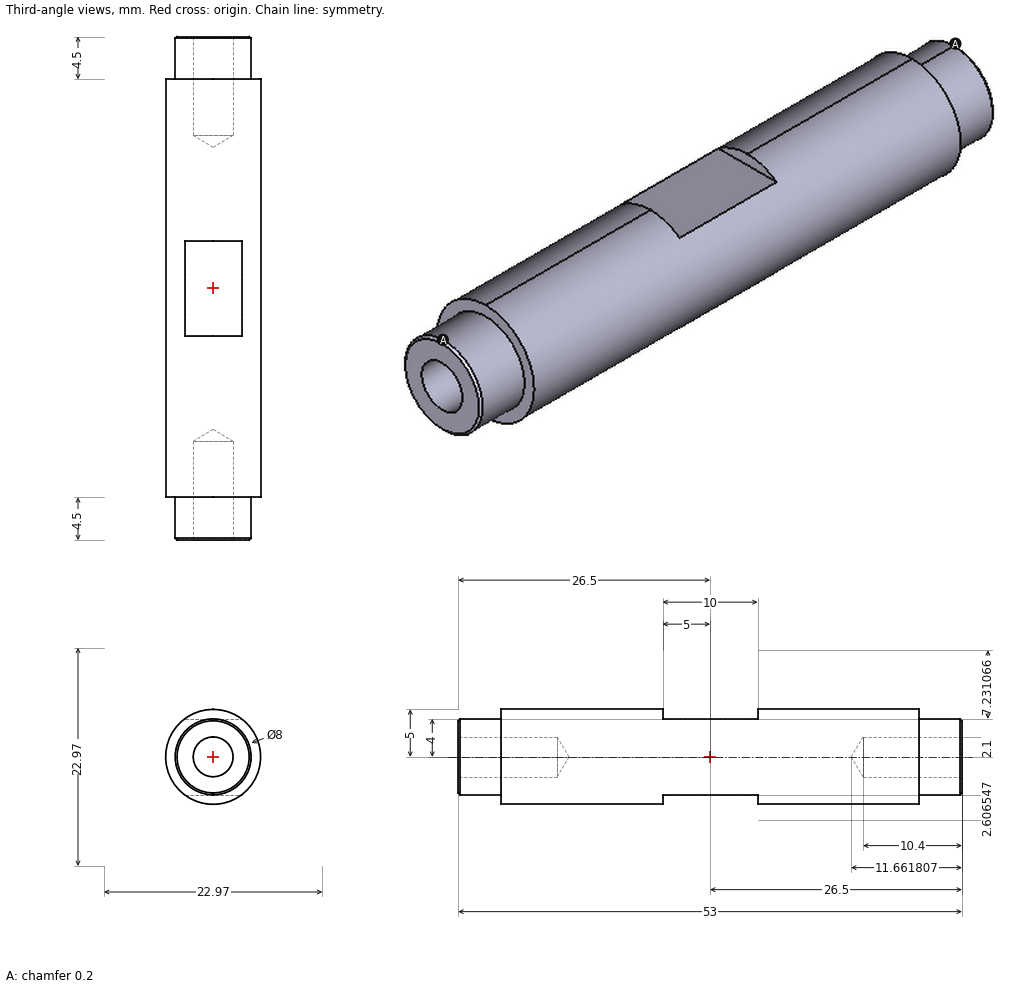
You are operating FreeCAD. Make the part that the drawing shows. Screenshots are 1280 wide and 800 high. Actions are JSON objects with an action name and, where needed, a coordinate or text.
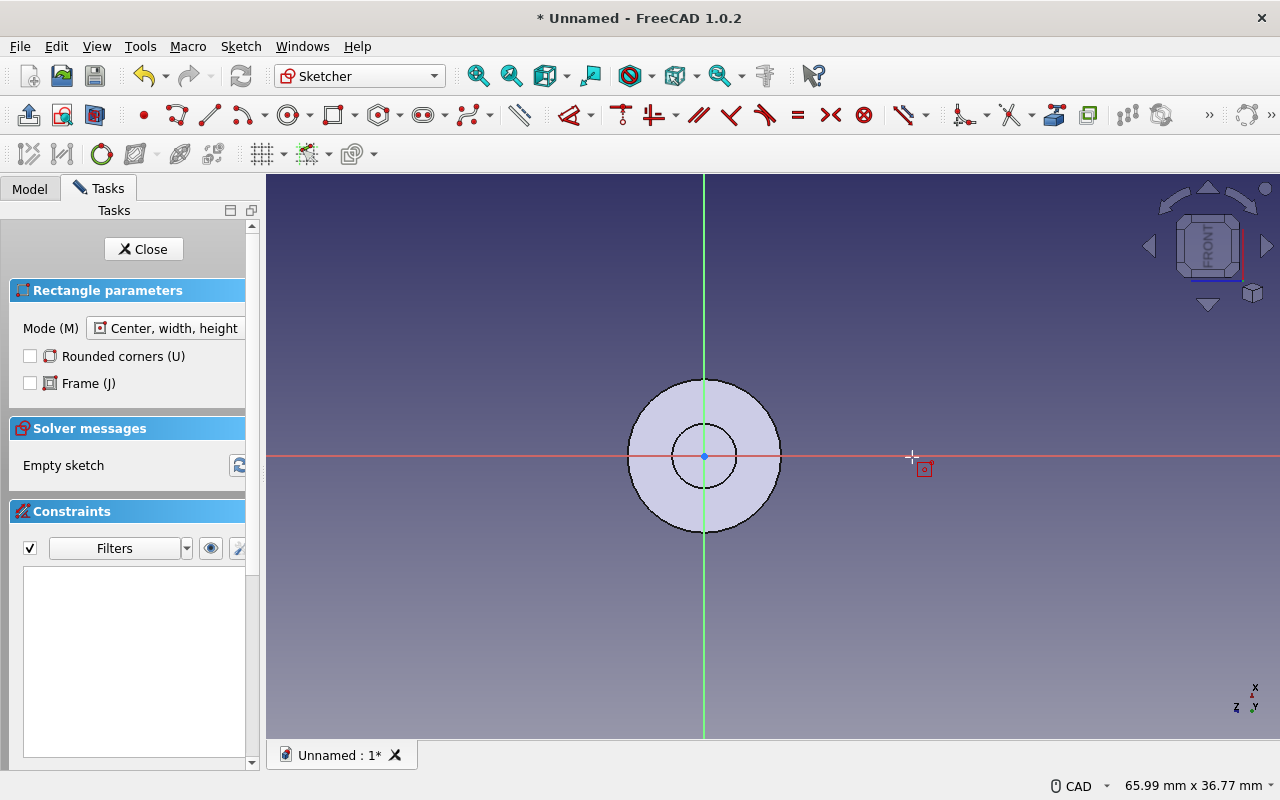
{"action": "left_click", "coordinate": [704, 456]}
{"action": "mouse_move", "coordinate": [881, 280]}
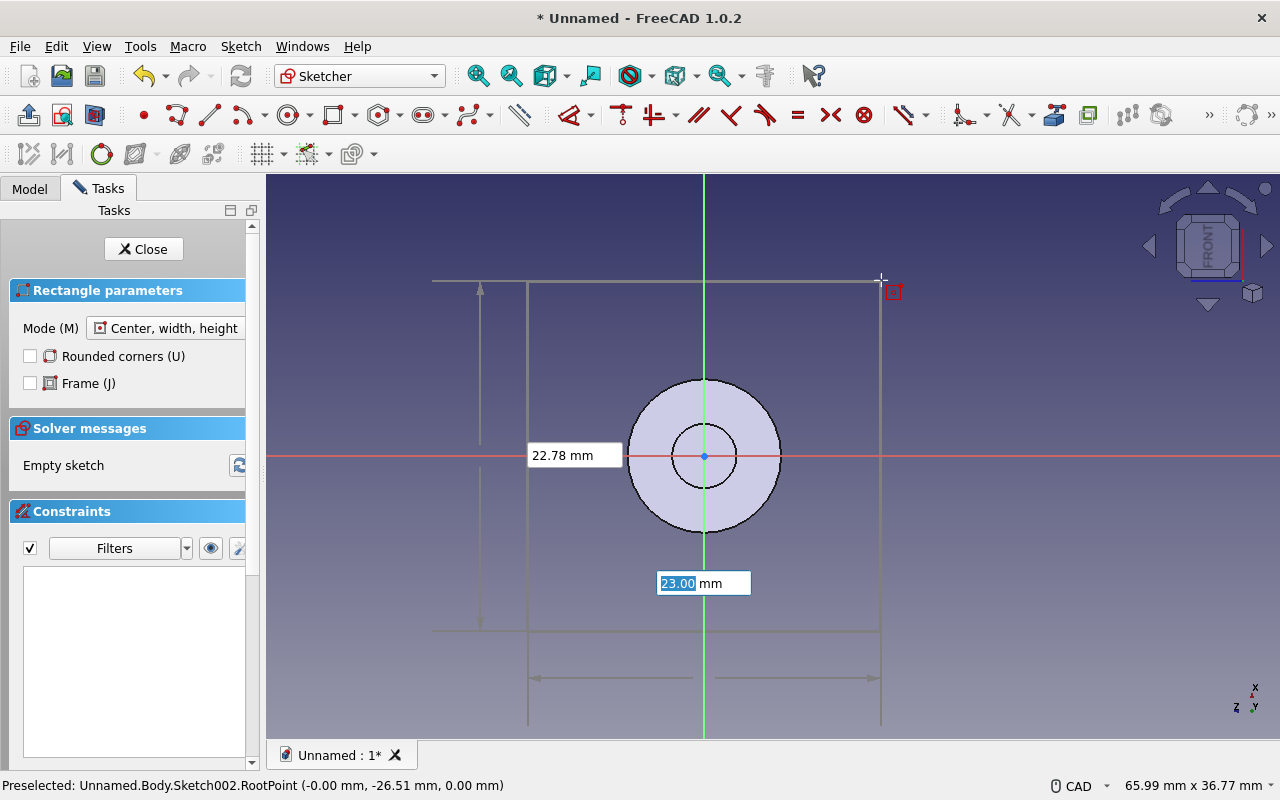
{"action": "type", "text": "22.97"}
{"action": "key", "text": "Tab"}
{"action": "type", "text": "22.97"}
{"action": "key", "text": "Return"}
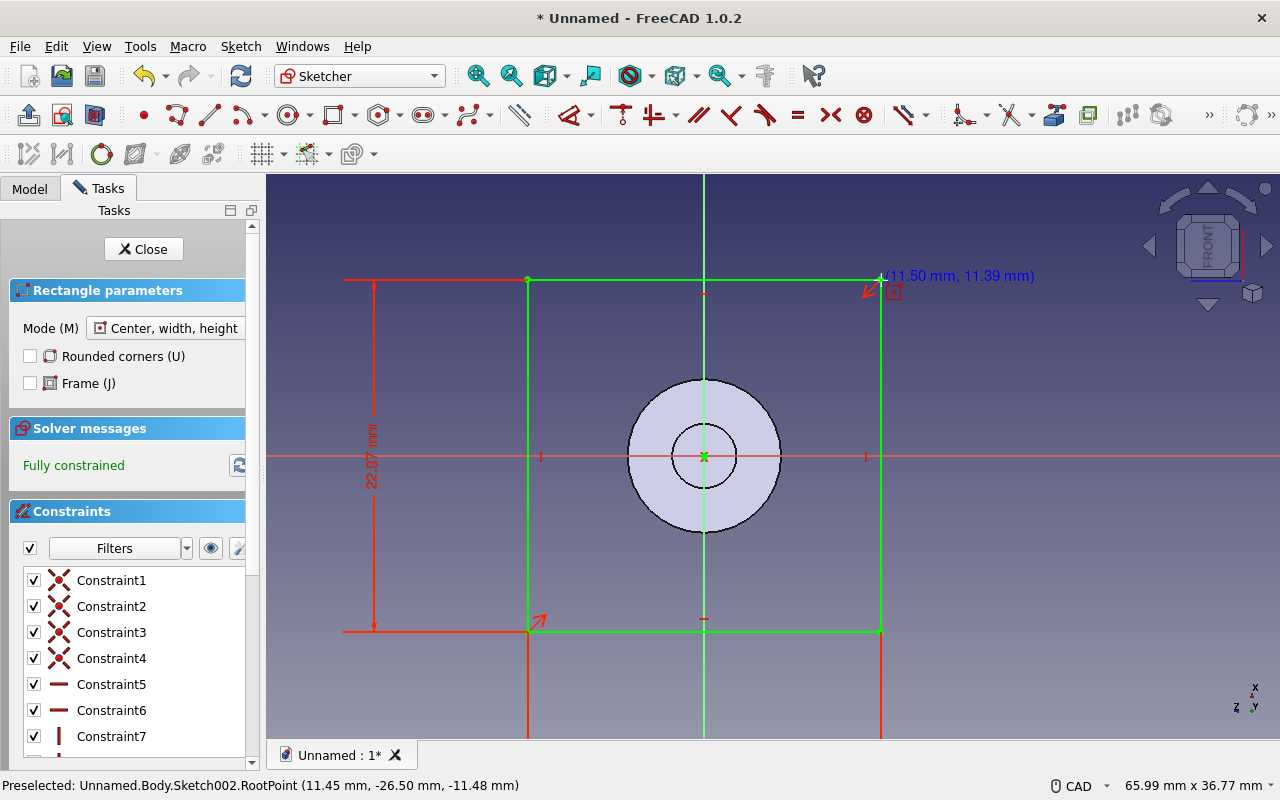
{"action": "left_click", "coordinate": [288, 116]}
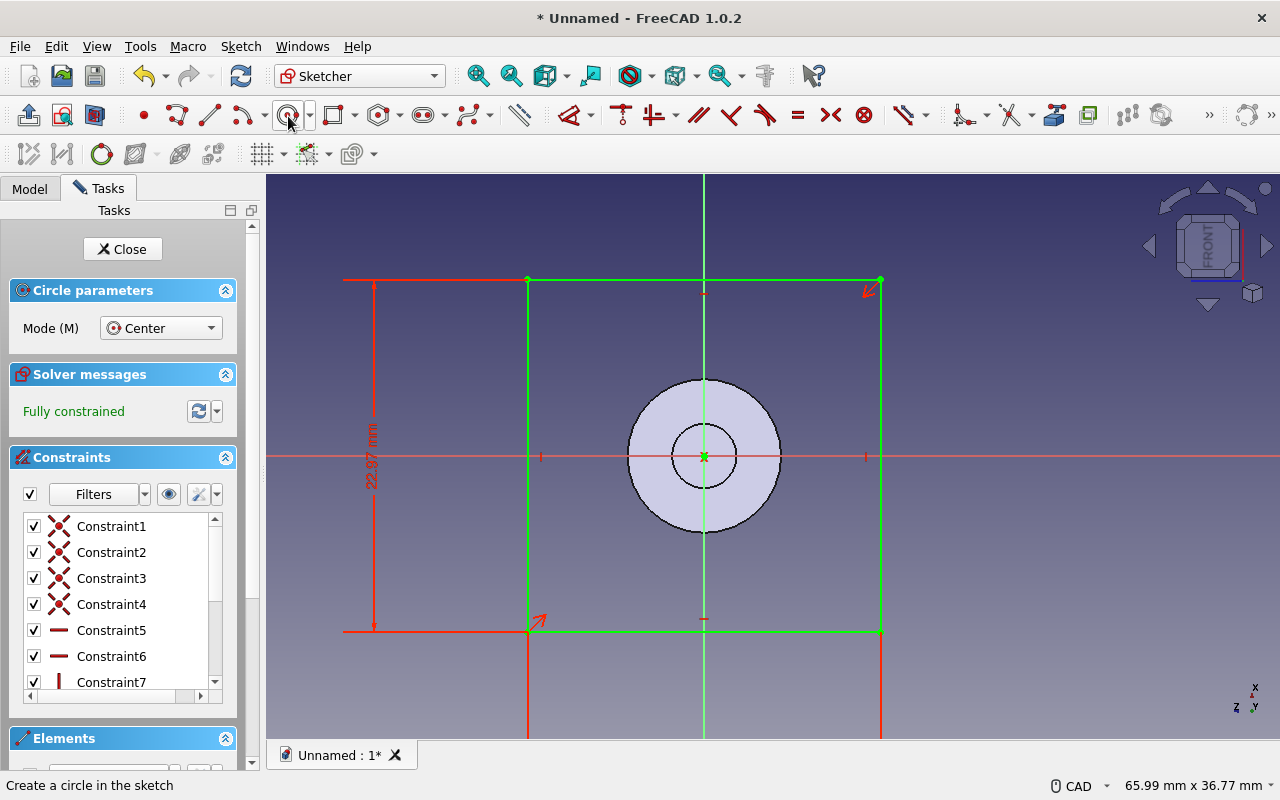
{"action": "left_click", "coordinate": [704, 456]}
{"action": "mouse_move", "coordinate": [748, 413]}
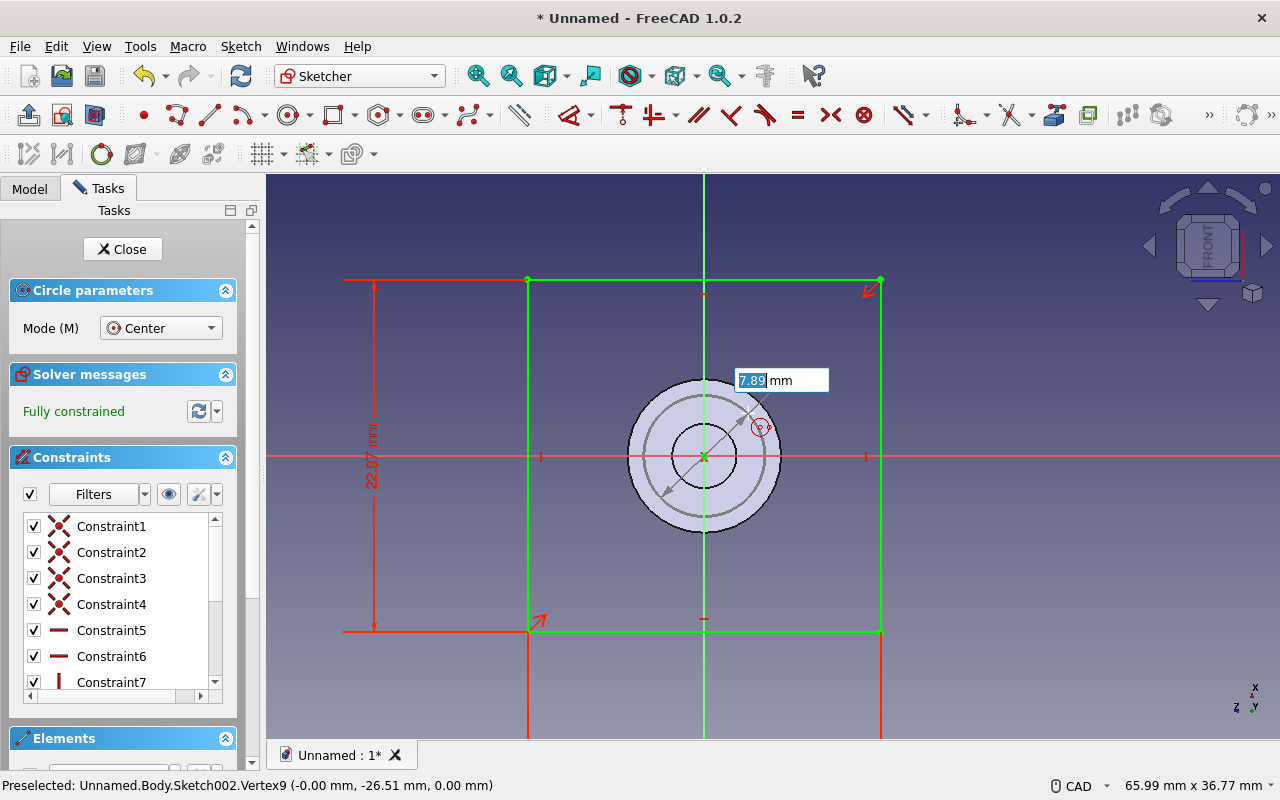
{"action": "type", "text": "8"}
{"action": "key", "text": "Return"}
{"action": "key", "text": "Escape"}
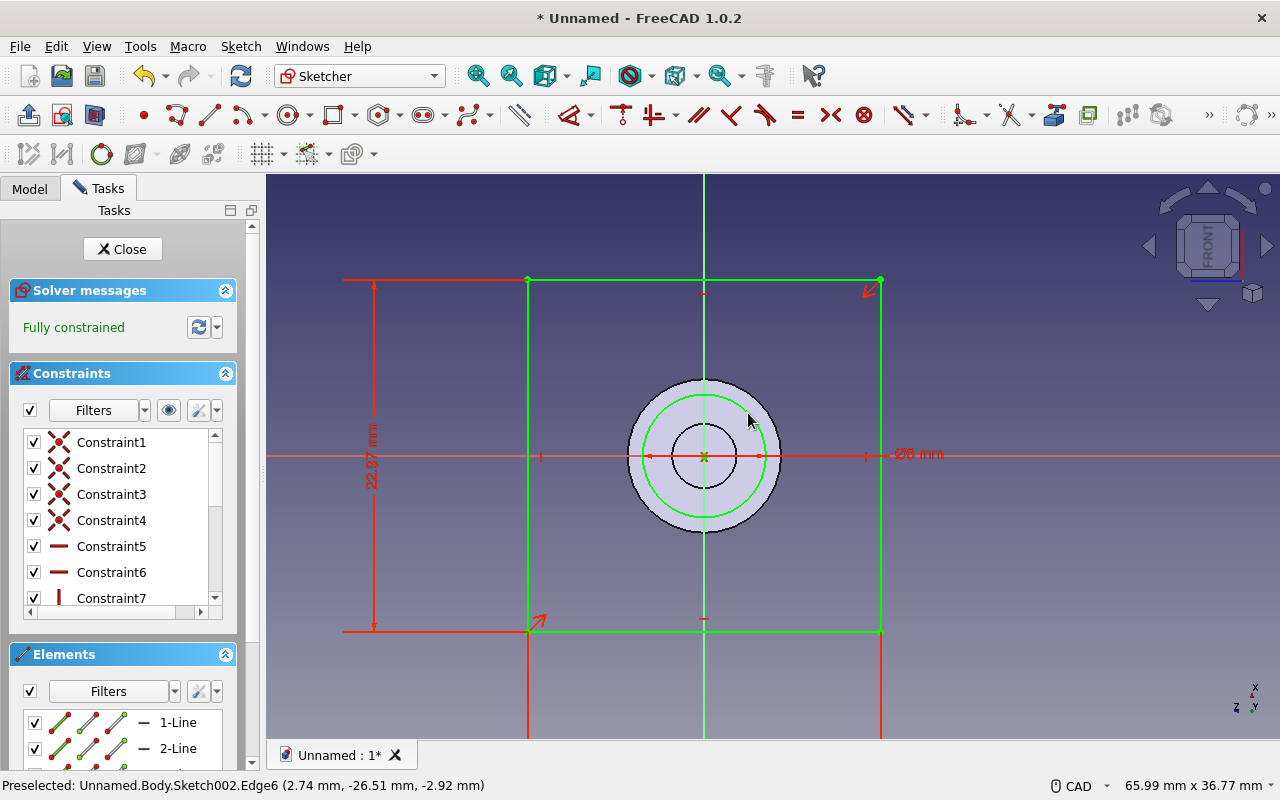
{"action": "left_click", "coordinate": [123, 249]}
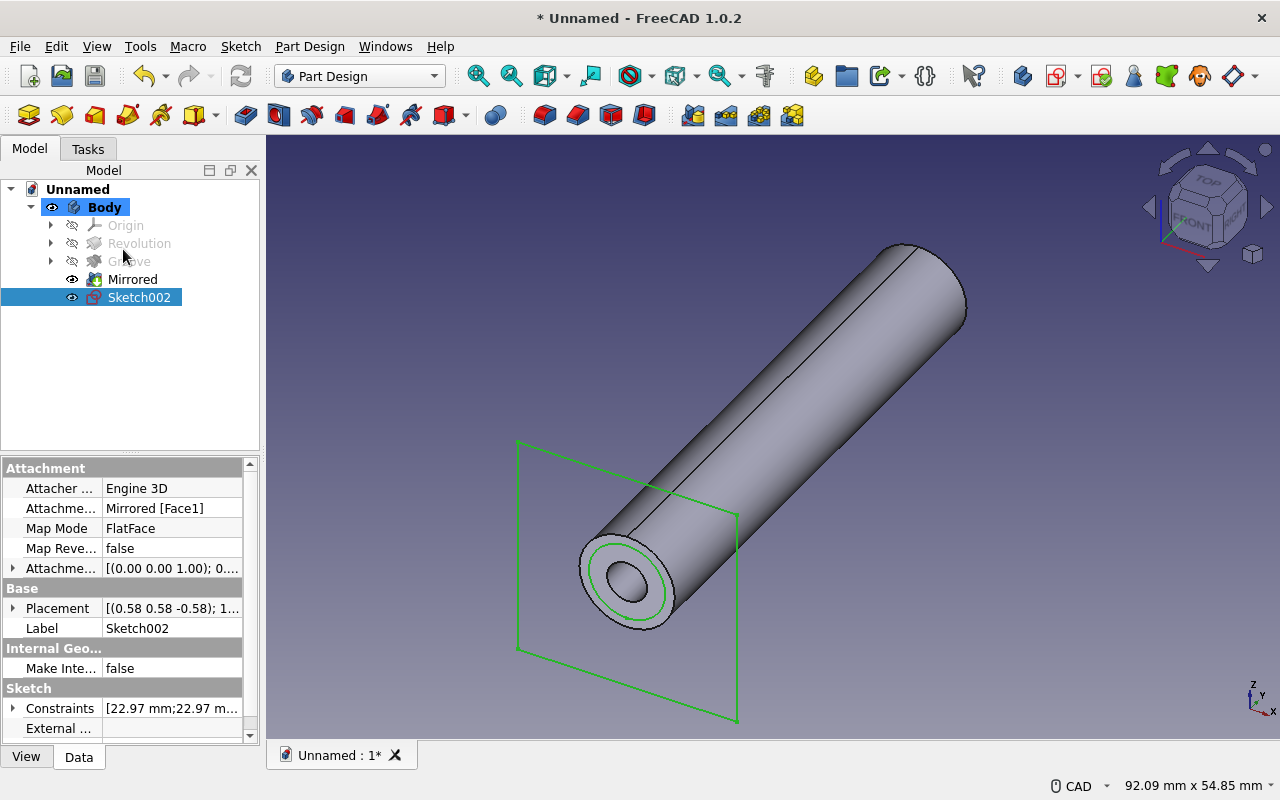
{"action": "left_click", "coordinate": [246, 116]}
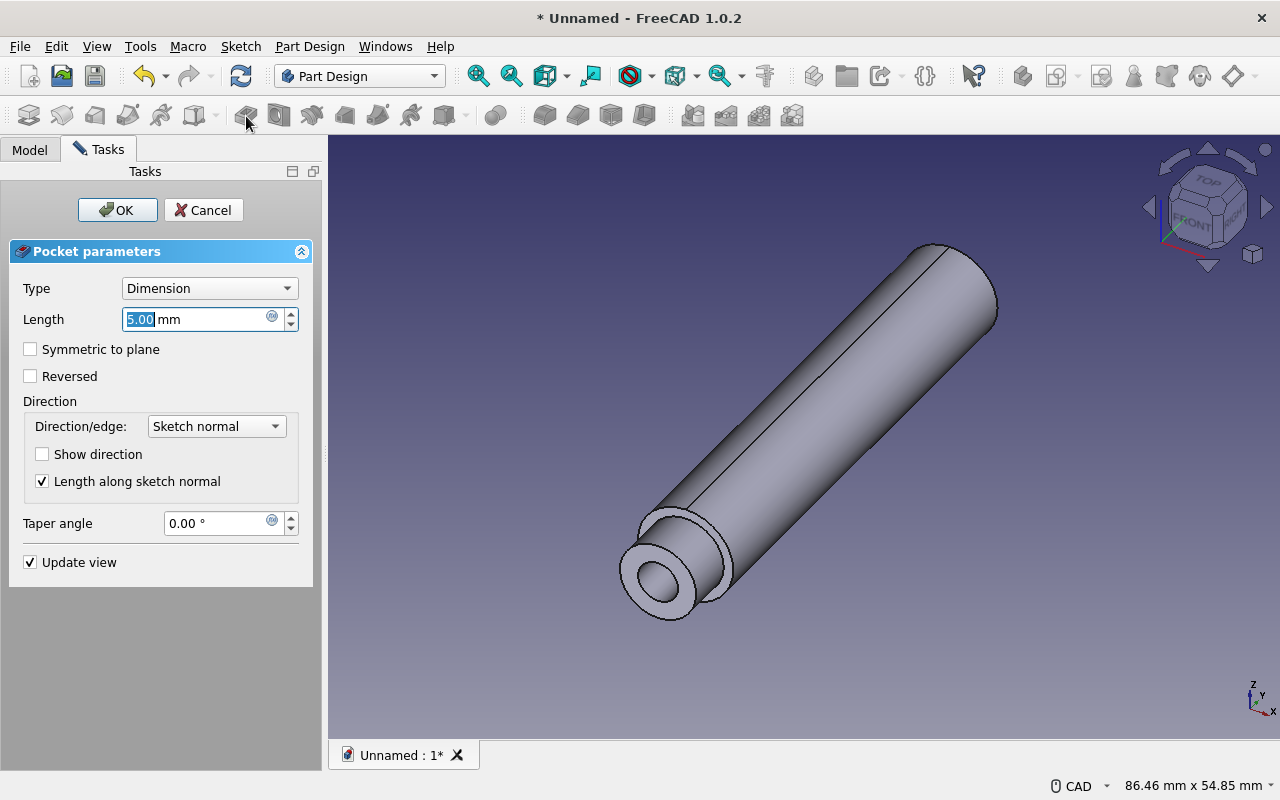
{"action": "type", "text": "4.5"}
{"action": "key", "text": "Tab"}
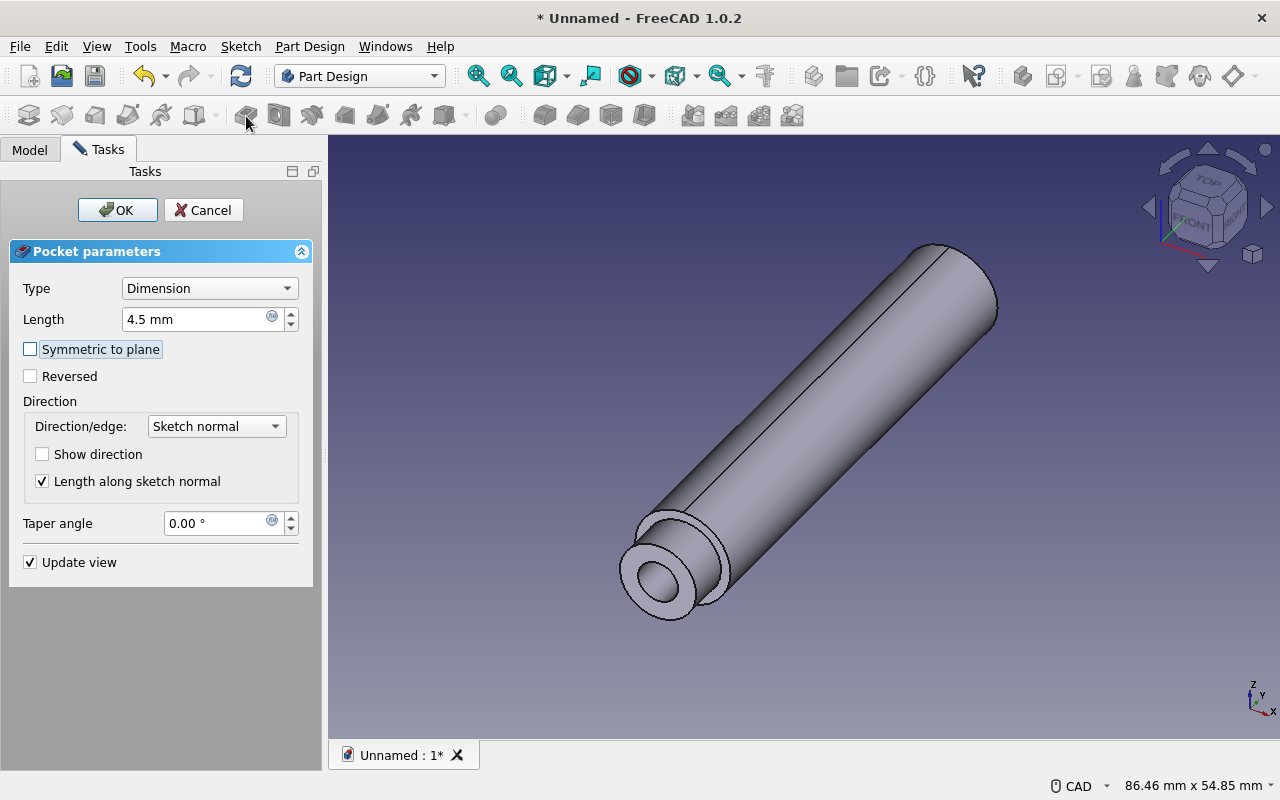
{"action": "left_click", "coordinate": [118, 210]}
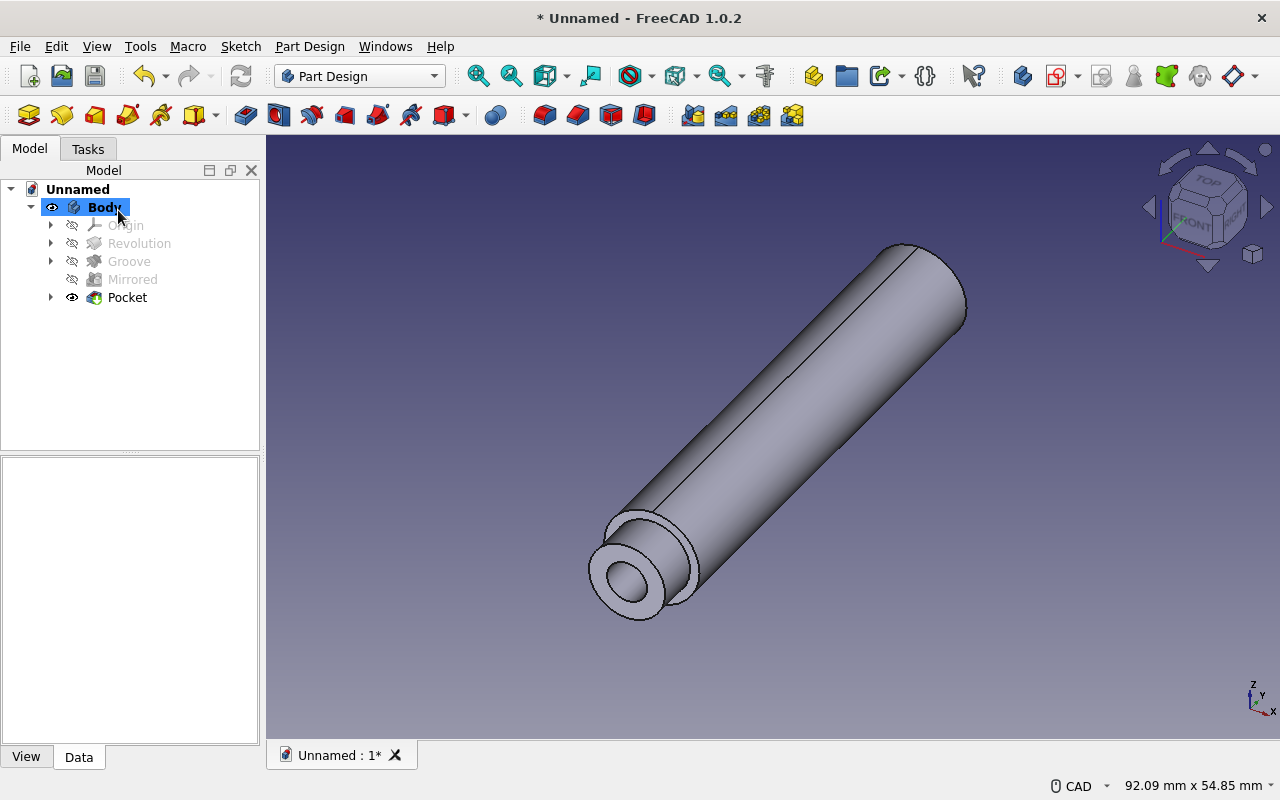
{"action": "key", "text": "4"}